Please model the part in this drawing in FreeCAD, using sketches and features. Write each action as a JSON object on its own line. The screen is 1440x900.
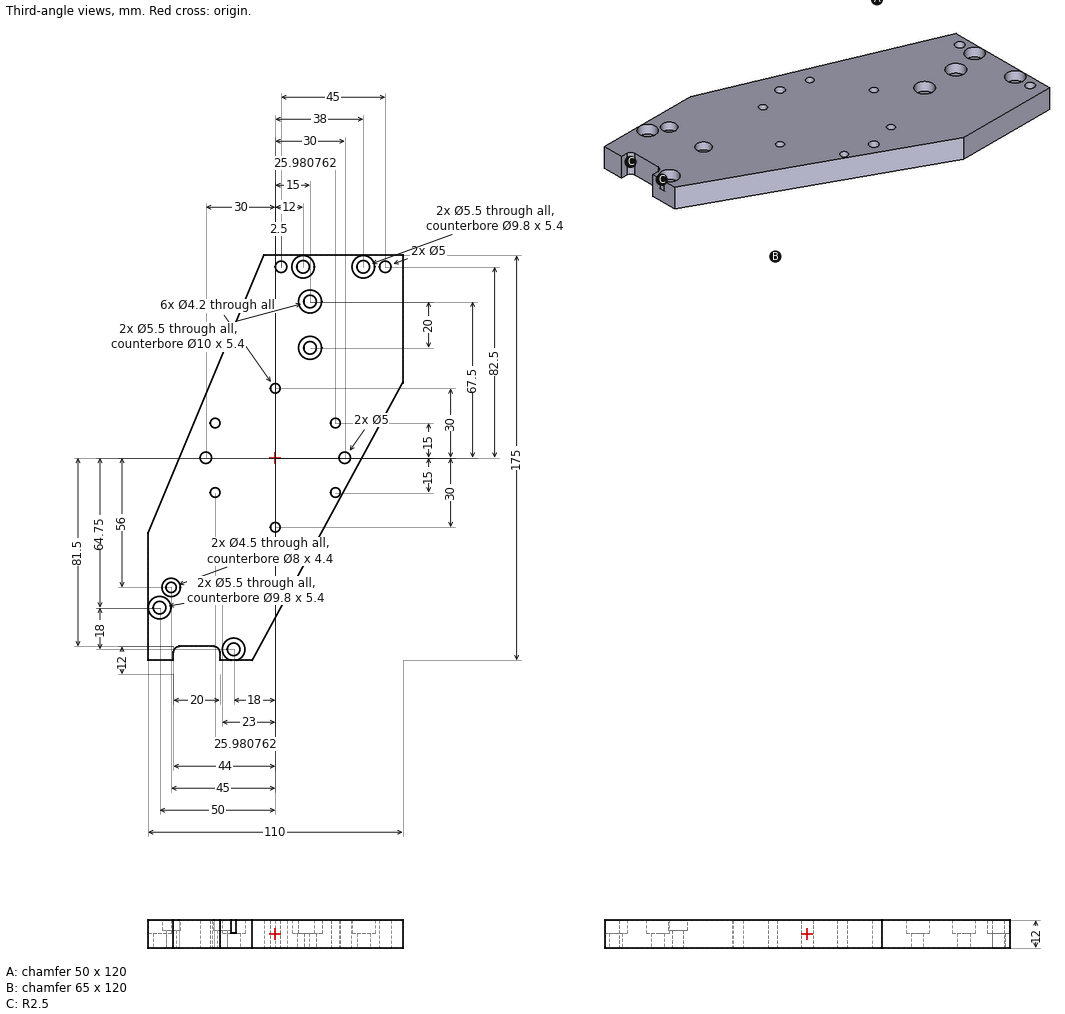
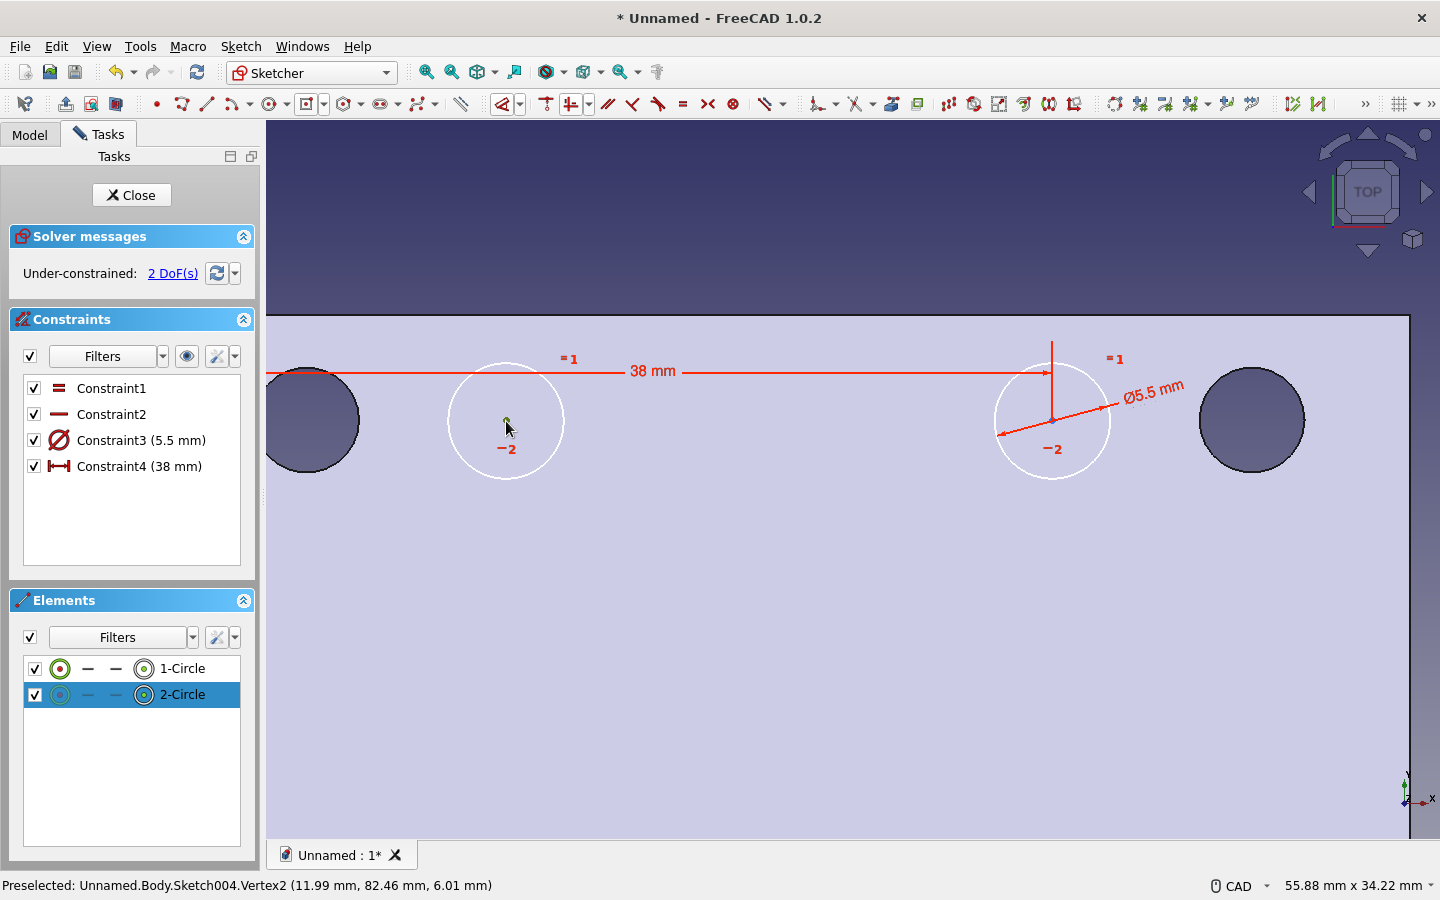
{"action": "key", "text": "l"}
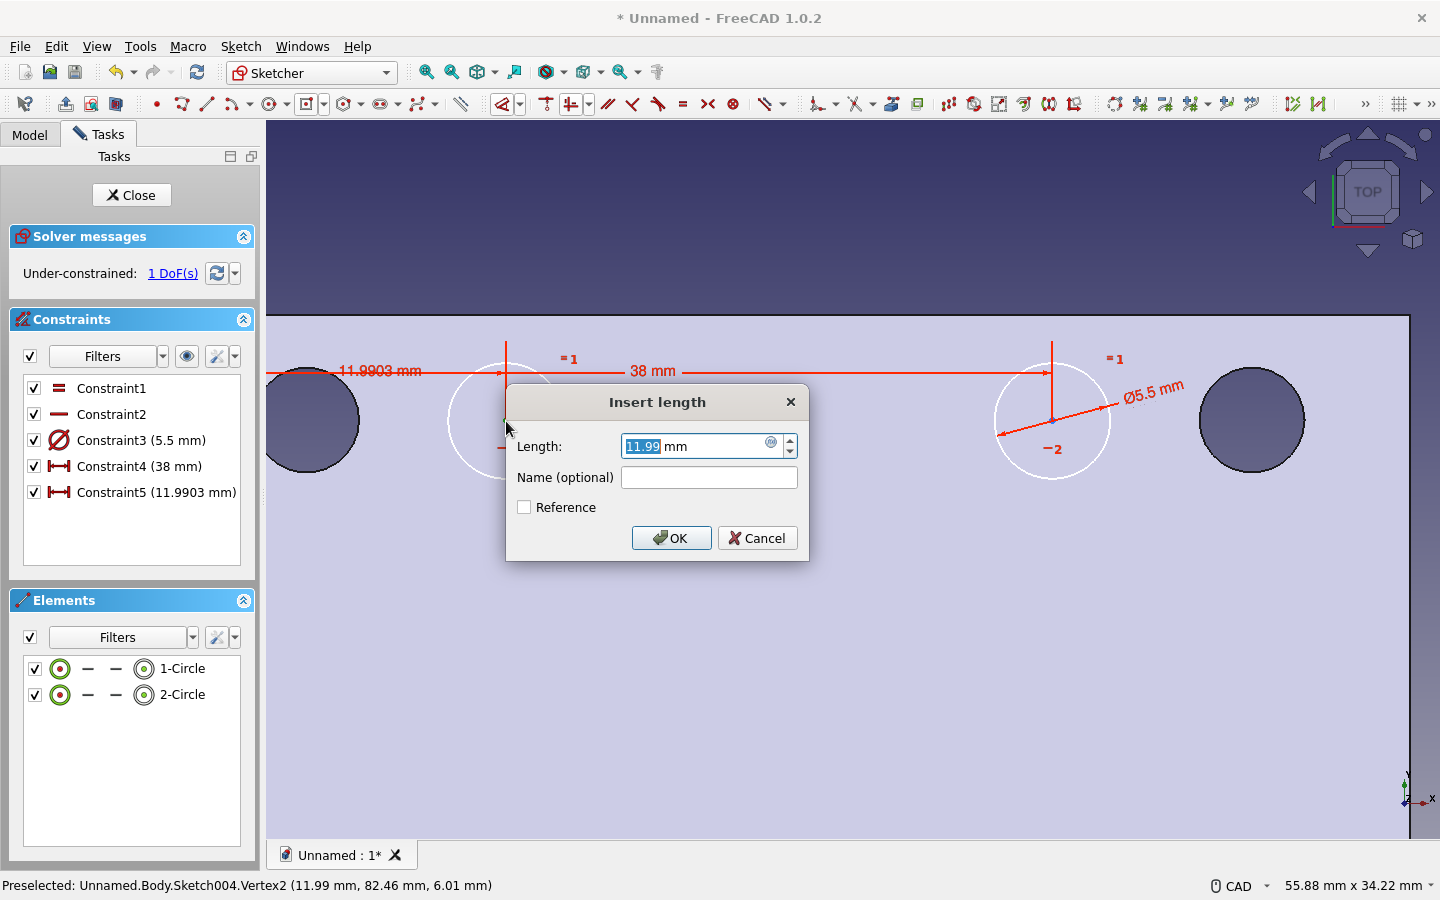
{"action": "type", "text": "12"}
{"action": "key", "text": "Return"}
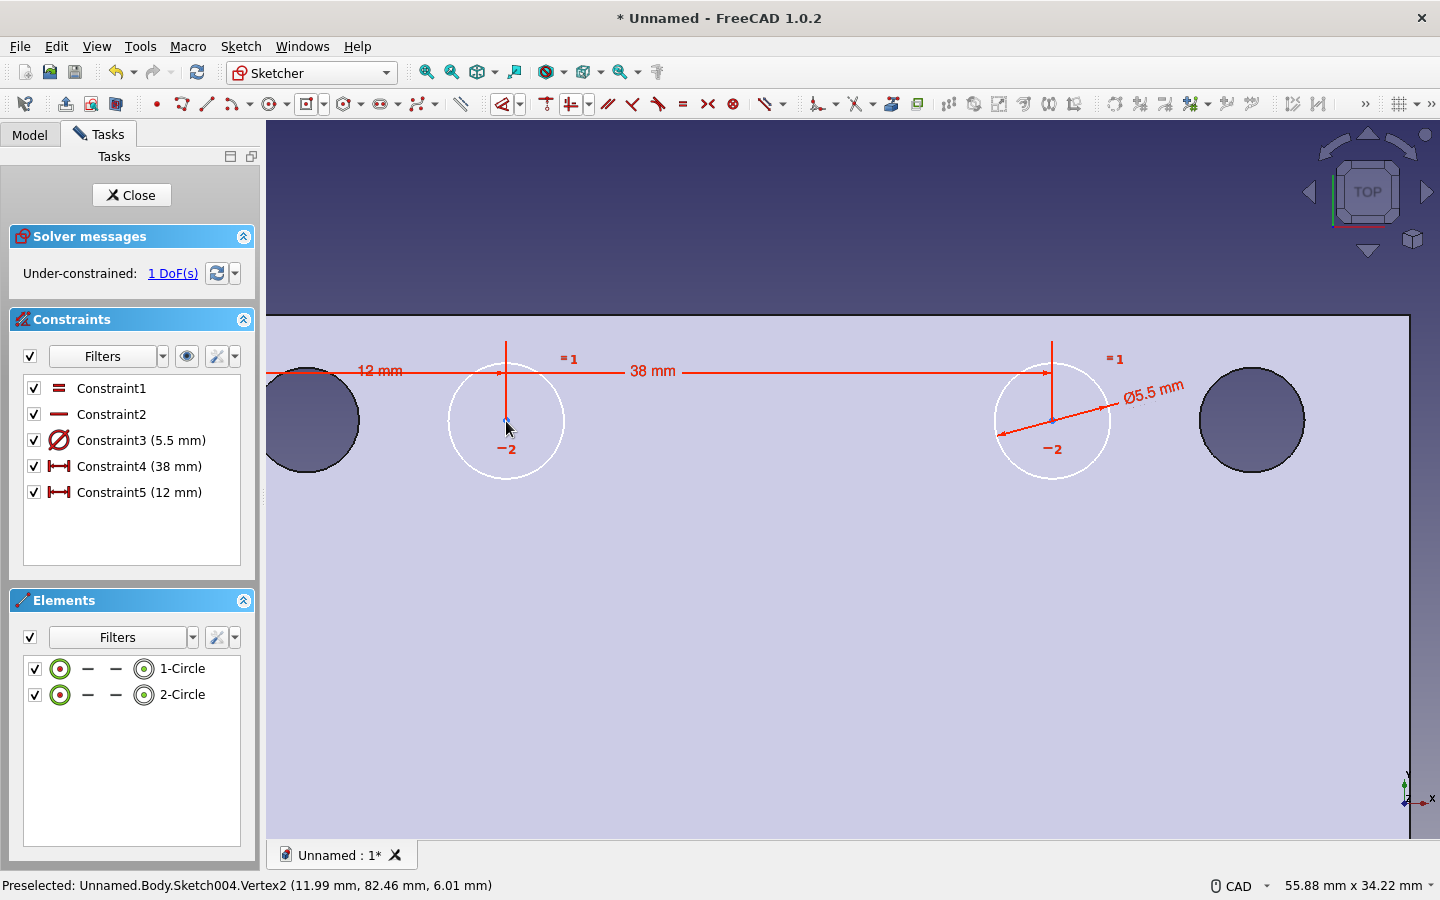
{"action": "left_click", "coordinate": [1052, 421]}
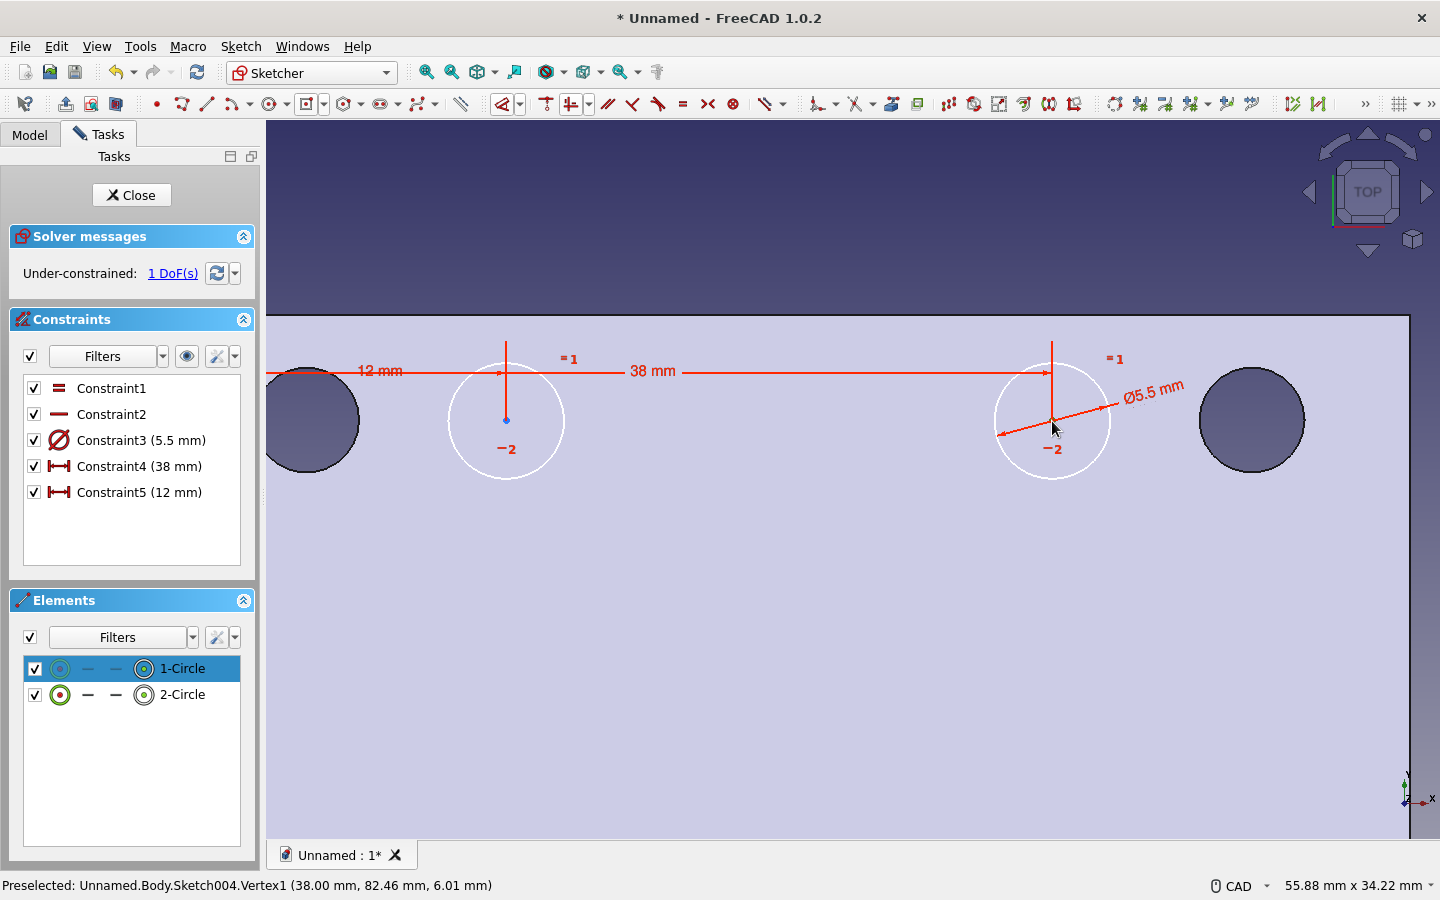
{"action": "left_click", "coordinate": [520, 104]}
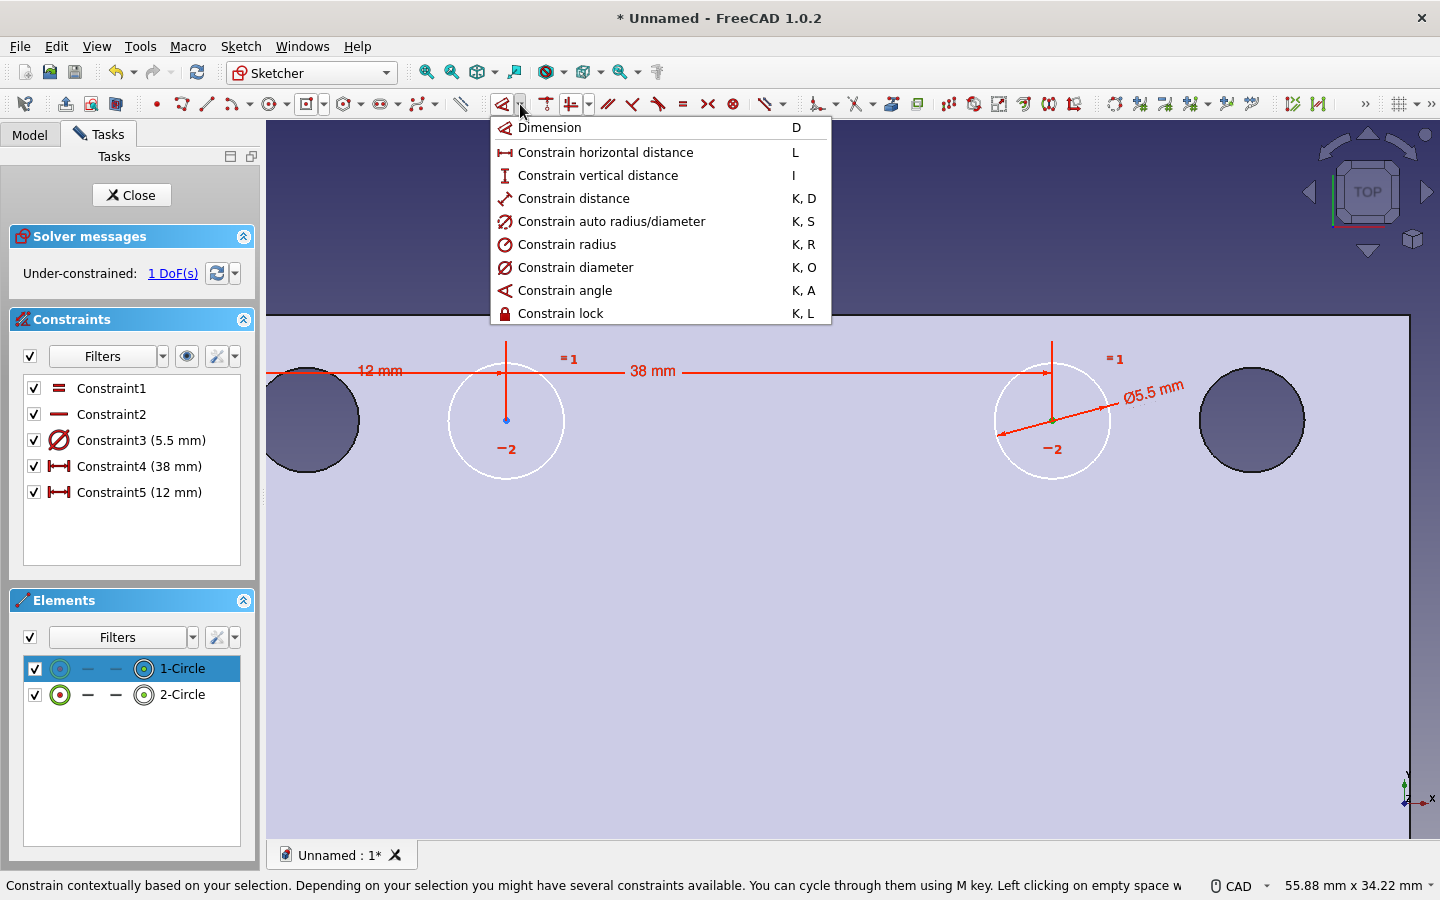
{"action": "left_click", "coordinate": [661, 176]}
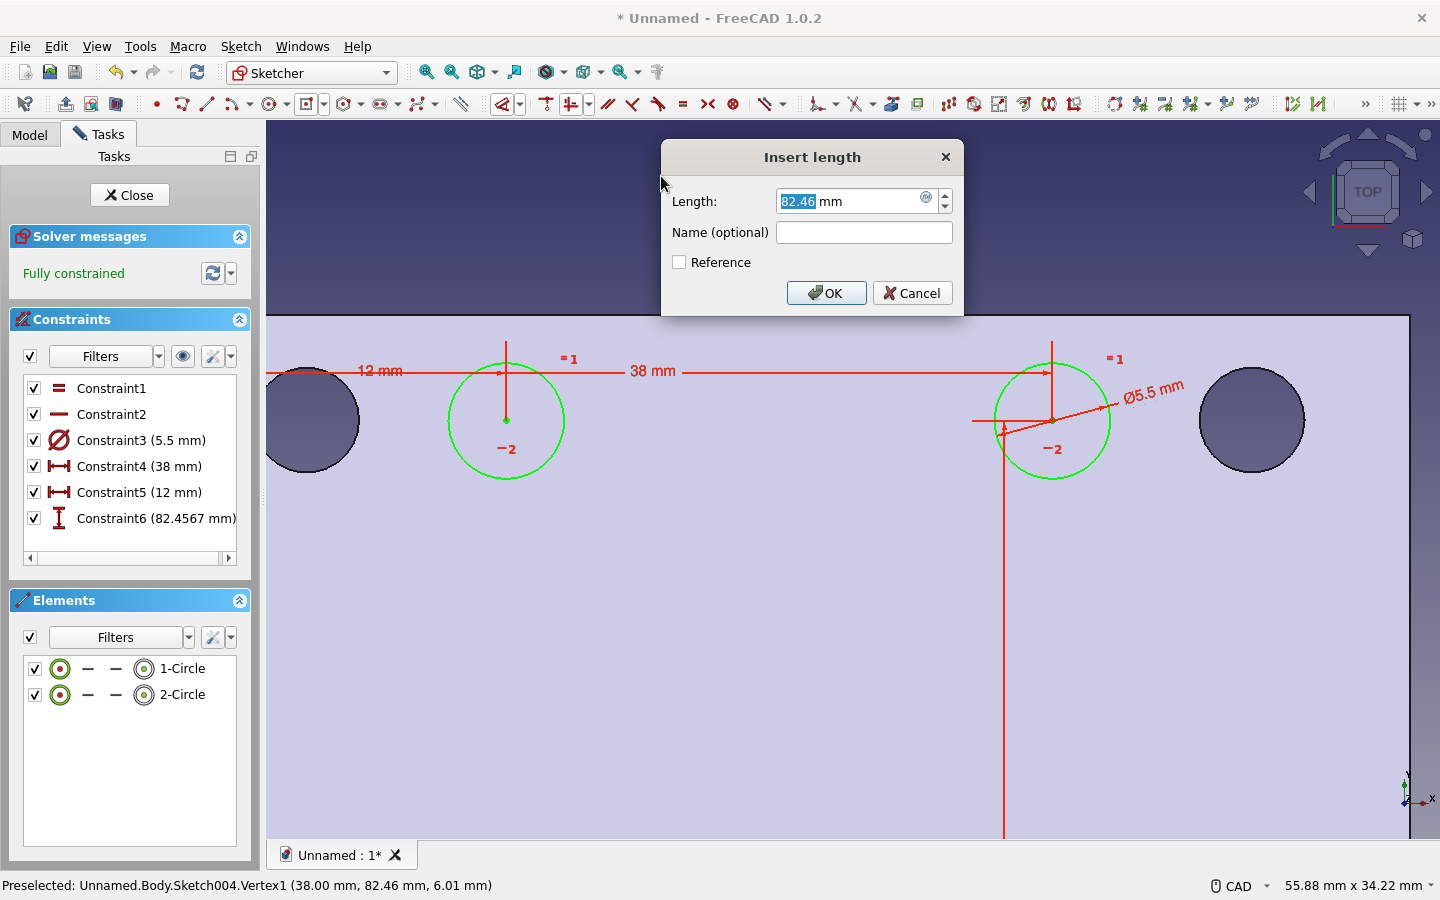
{"action": "type", "text": "82.5"}
{"action": "key", "text": "Return"}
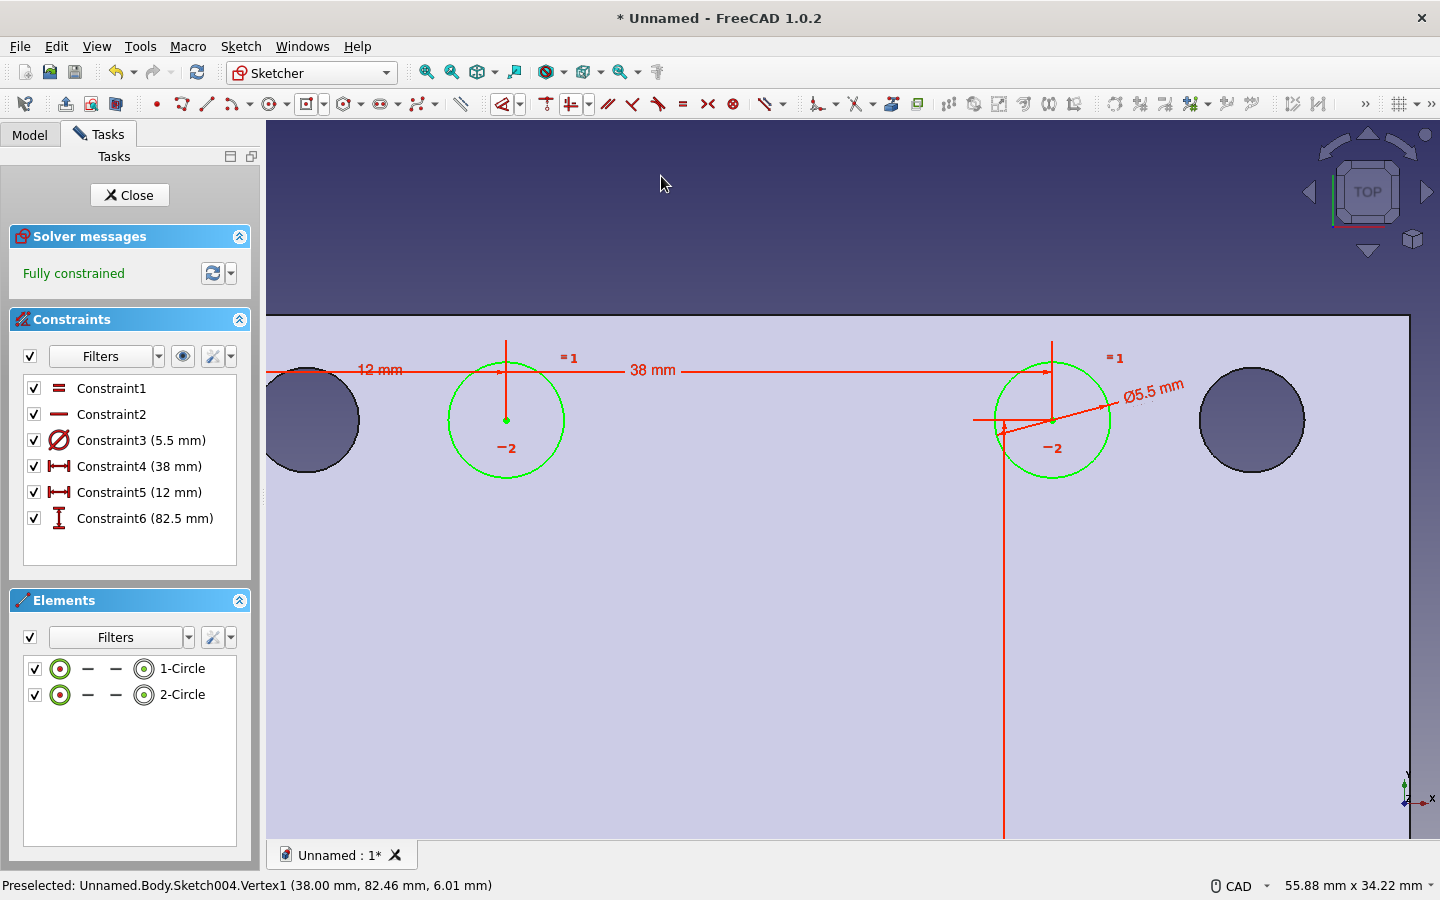
{"action": "left_click", "coordinate": [130, 195]}